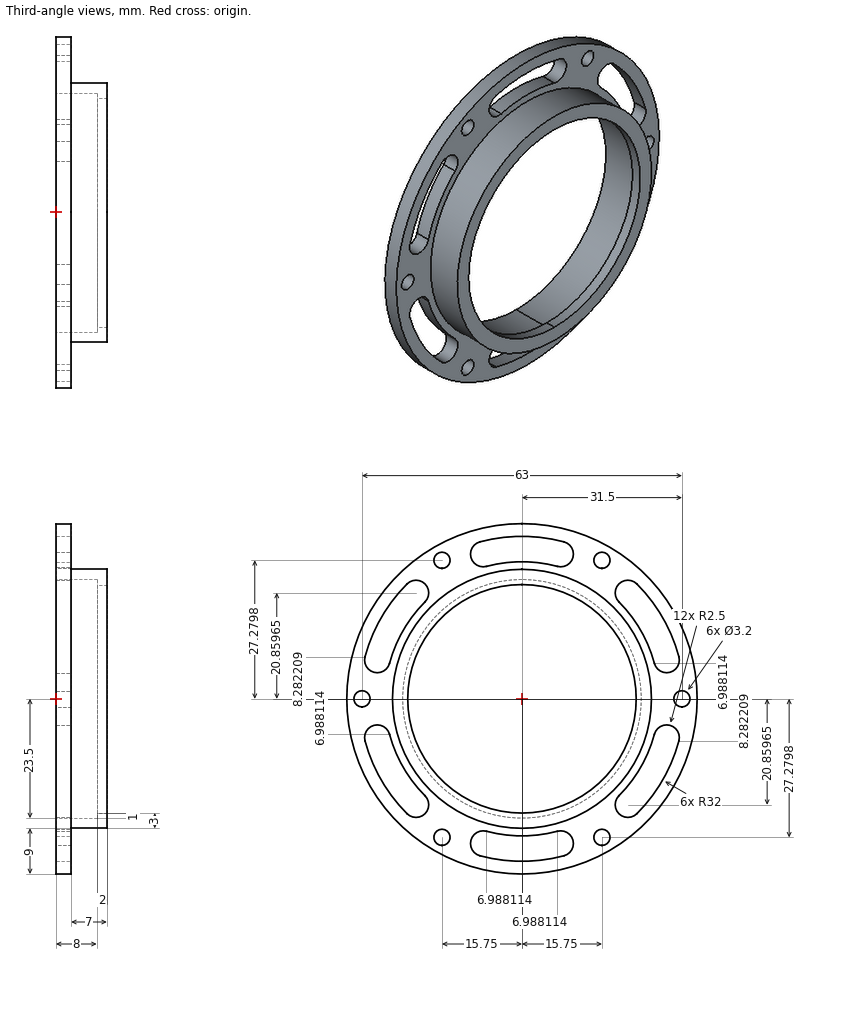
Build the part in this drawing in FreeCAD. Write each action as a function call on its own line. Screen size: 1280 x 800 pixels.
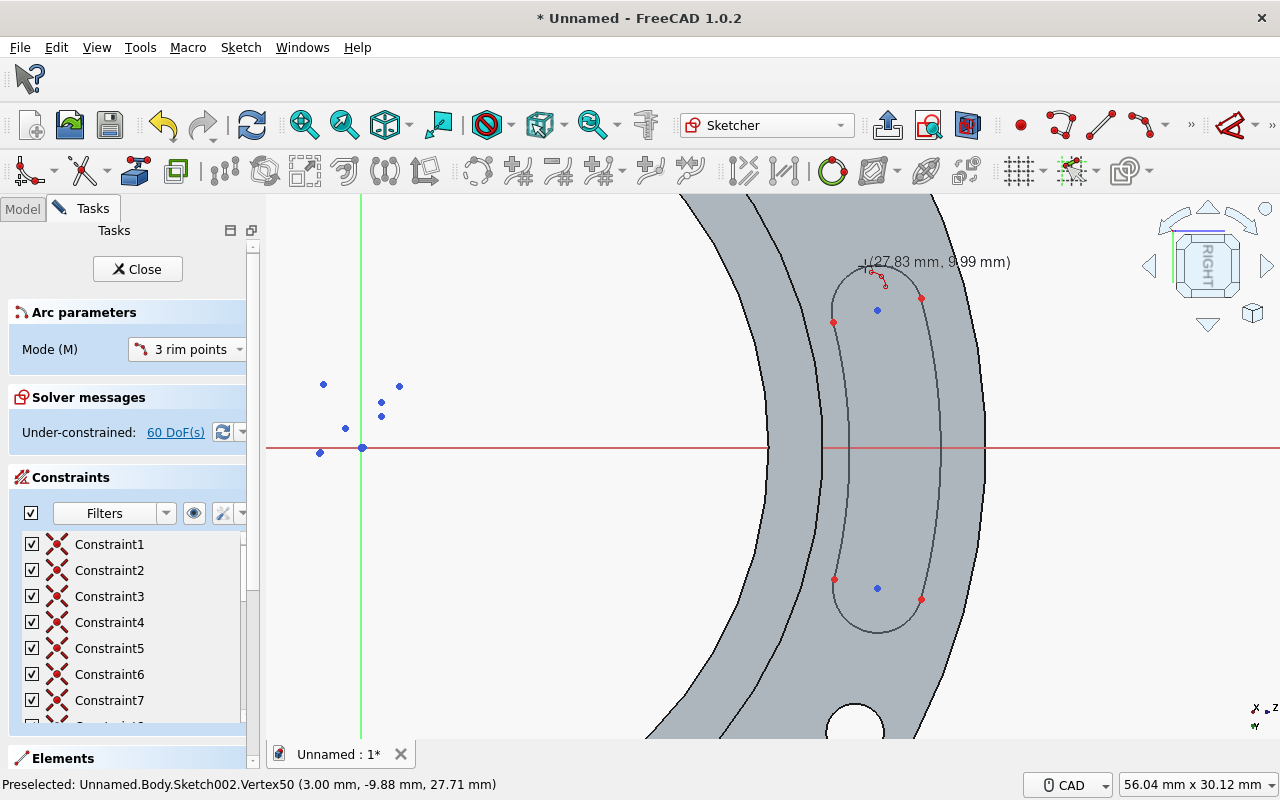
scroll(852, 475, down, 6)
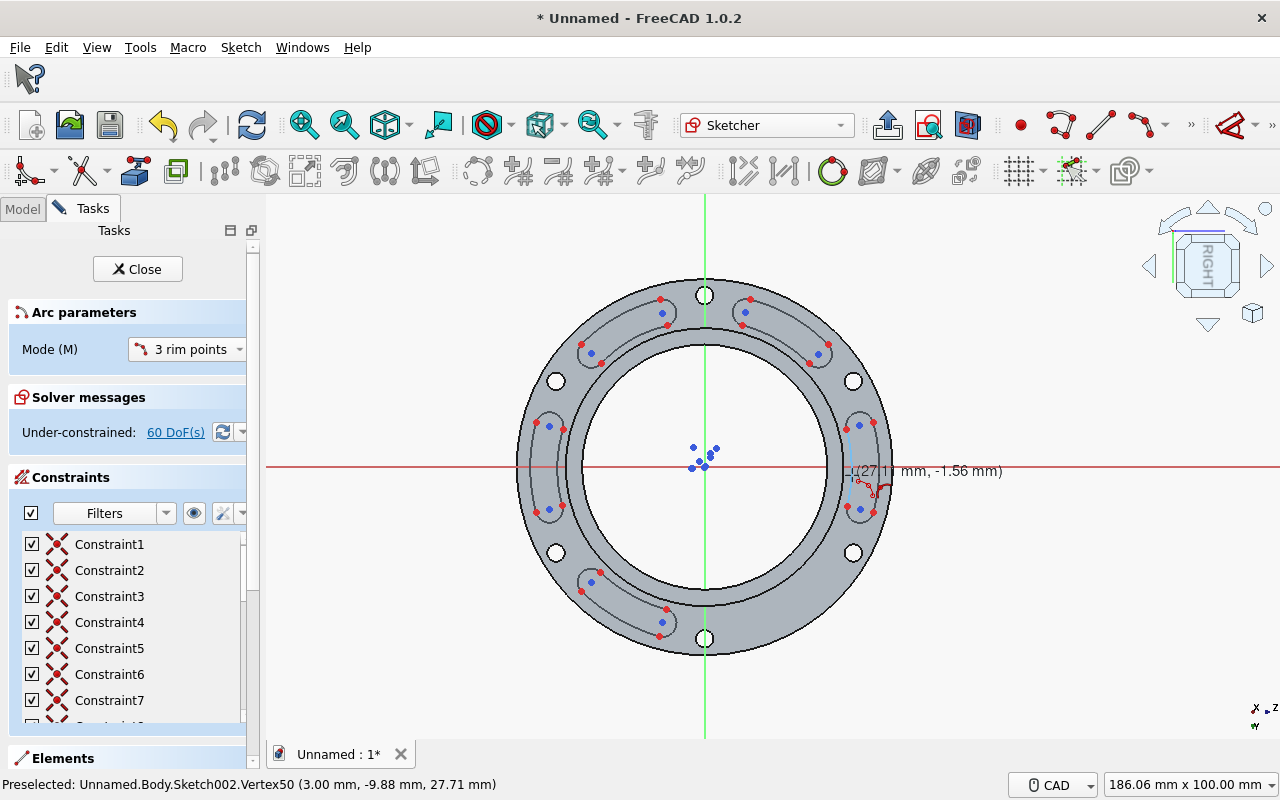
click(809, 571)
click(743, 609)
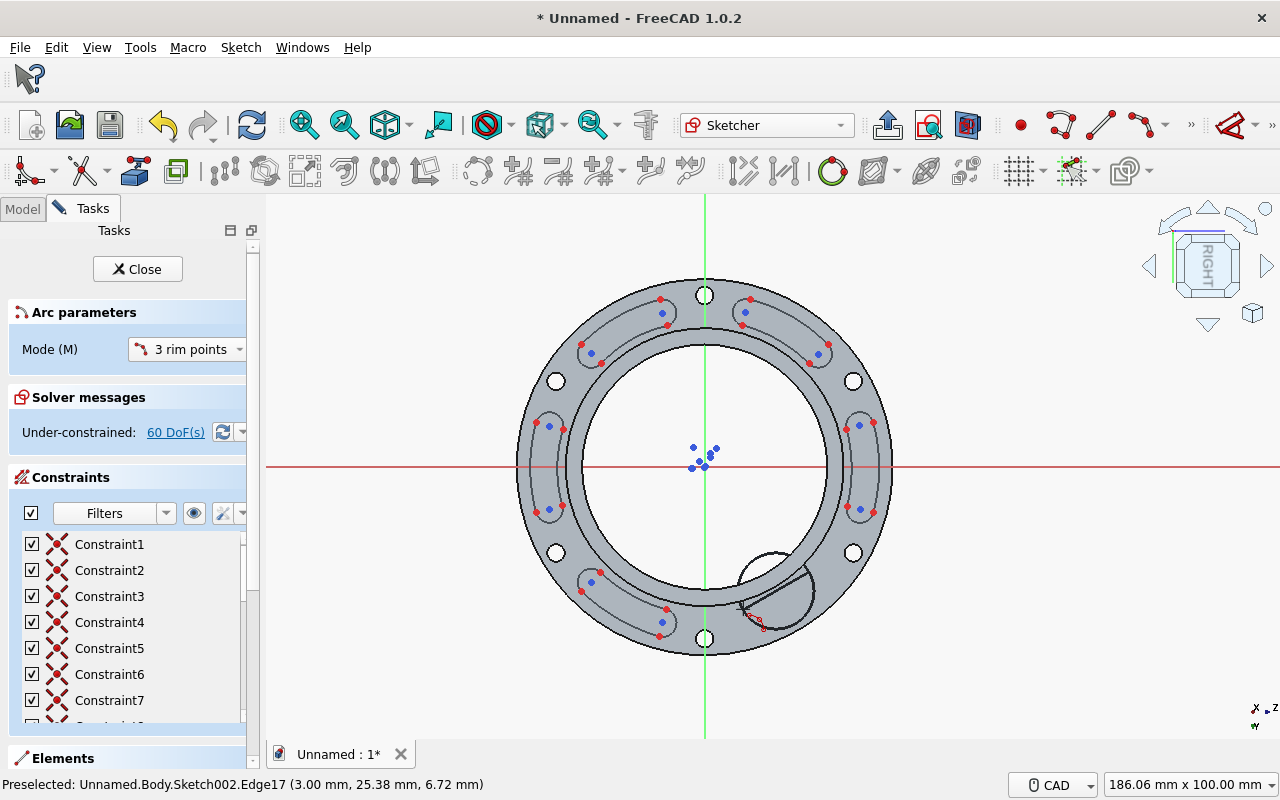
scroll(778, 595, up, 6)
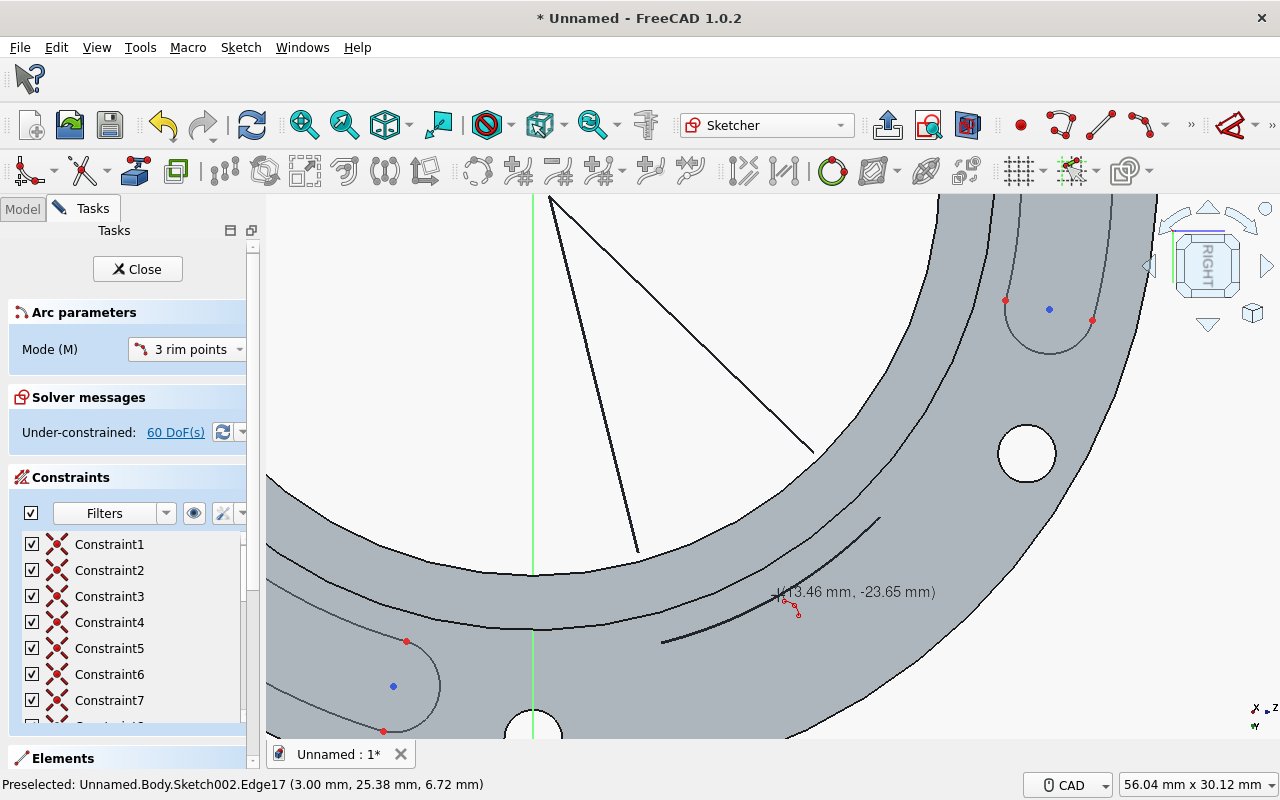
click(778, 592)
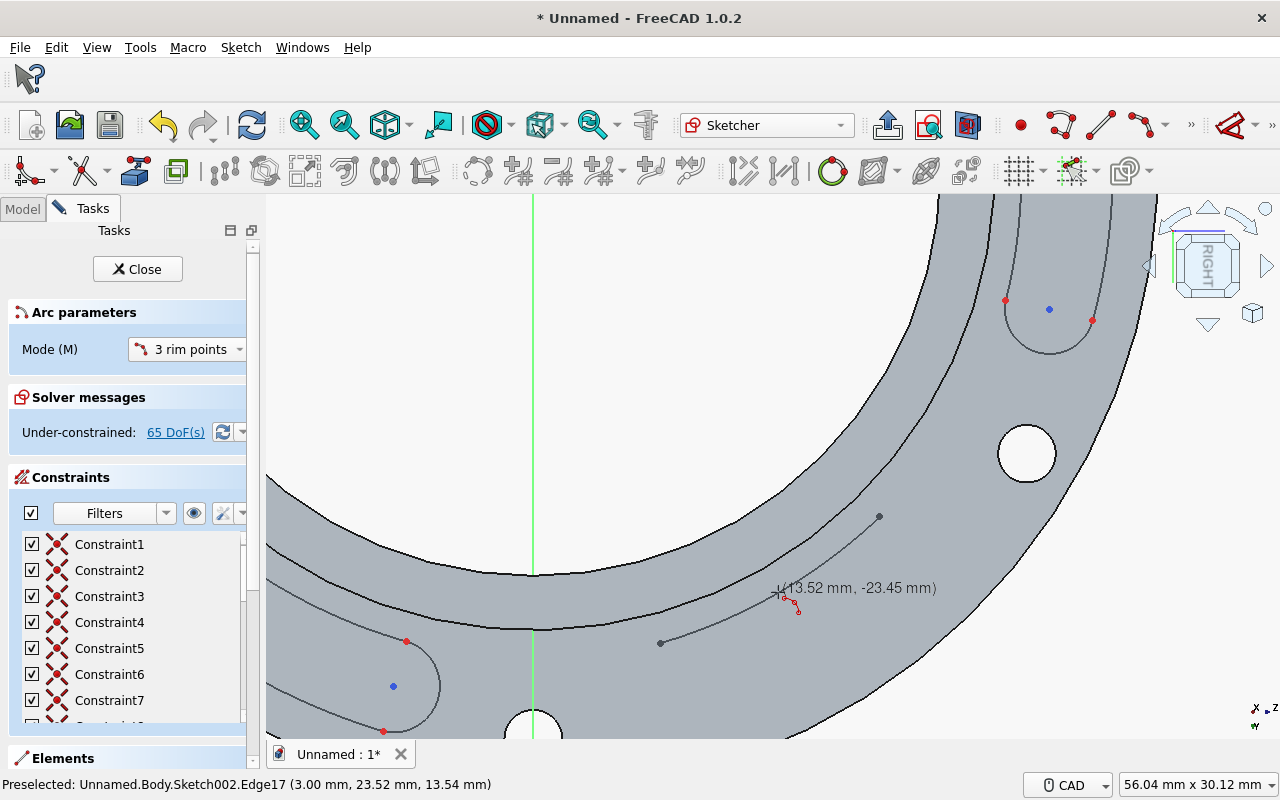
click(661, 643)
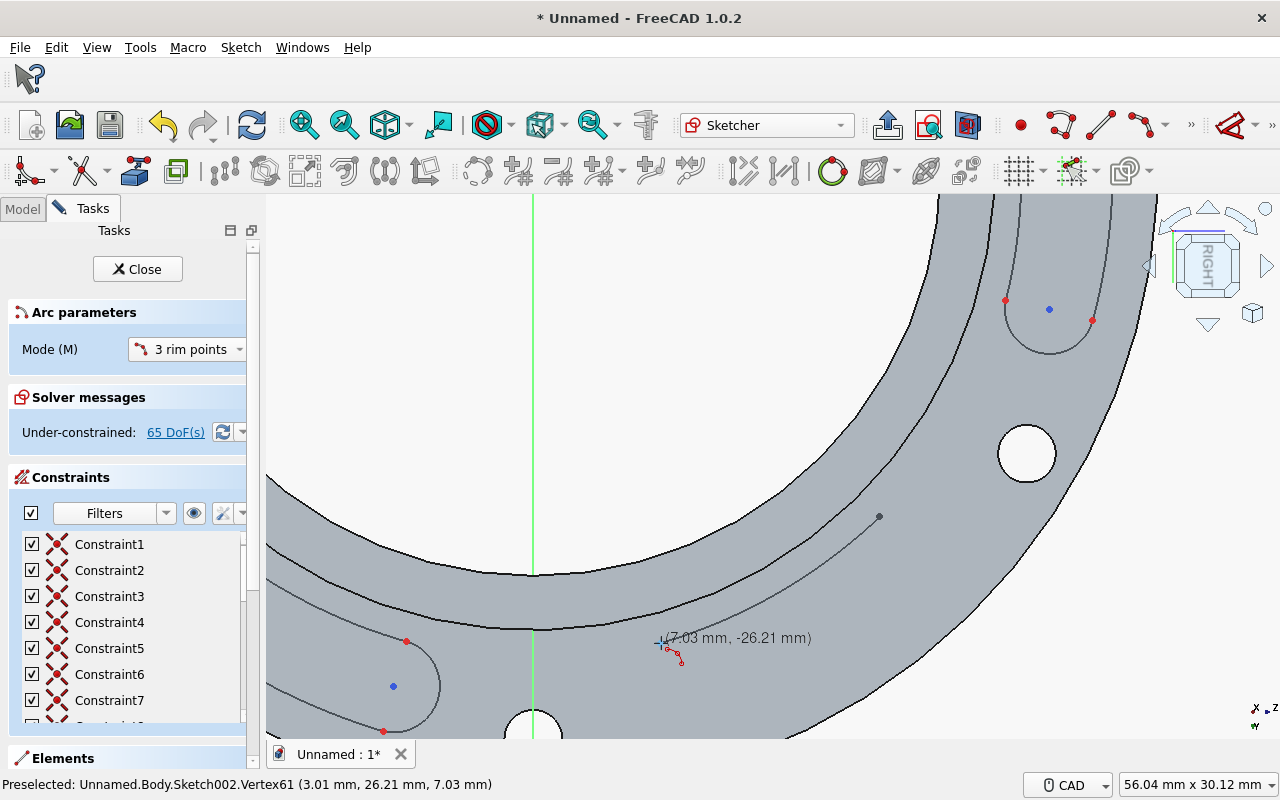
scroll(778, 595, down, 6)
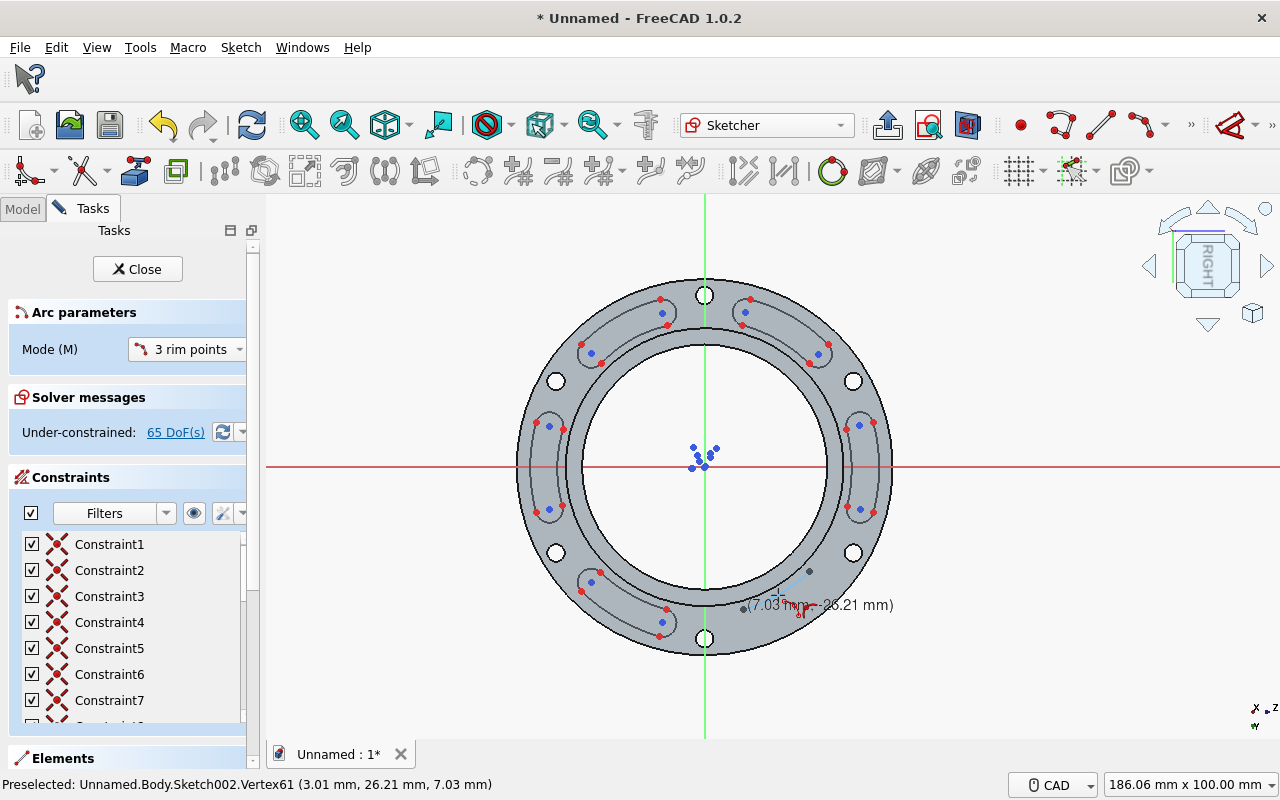
click(750, 636)
click(733, 626)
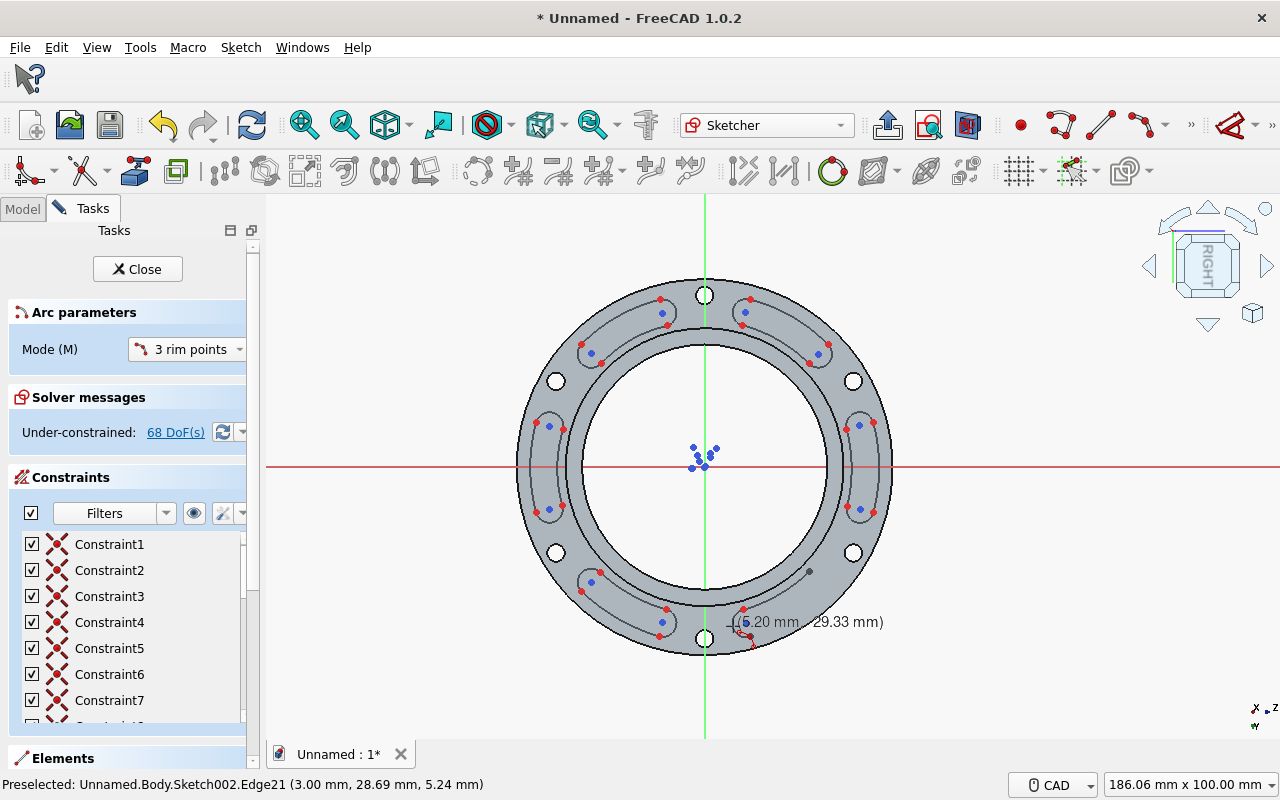
click(750, 637)
click(828, 590)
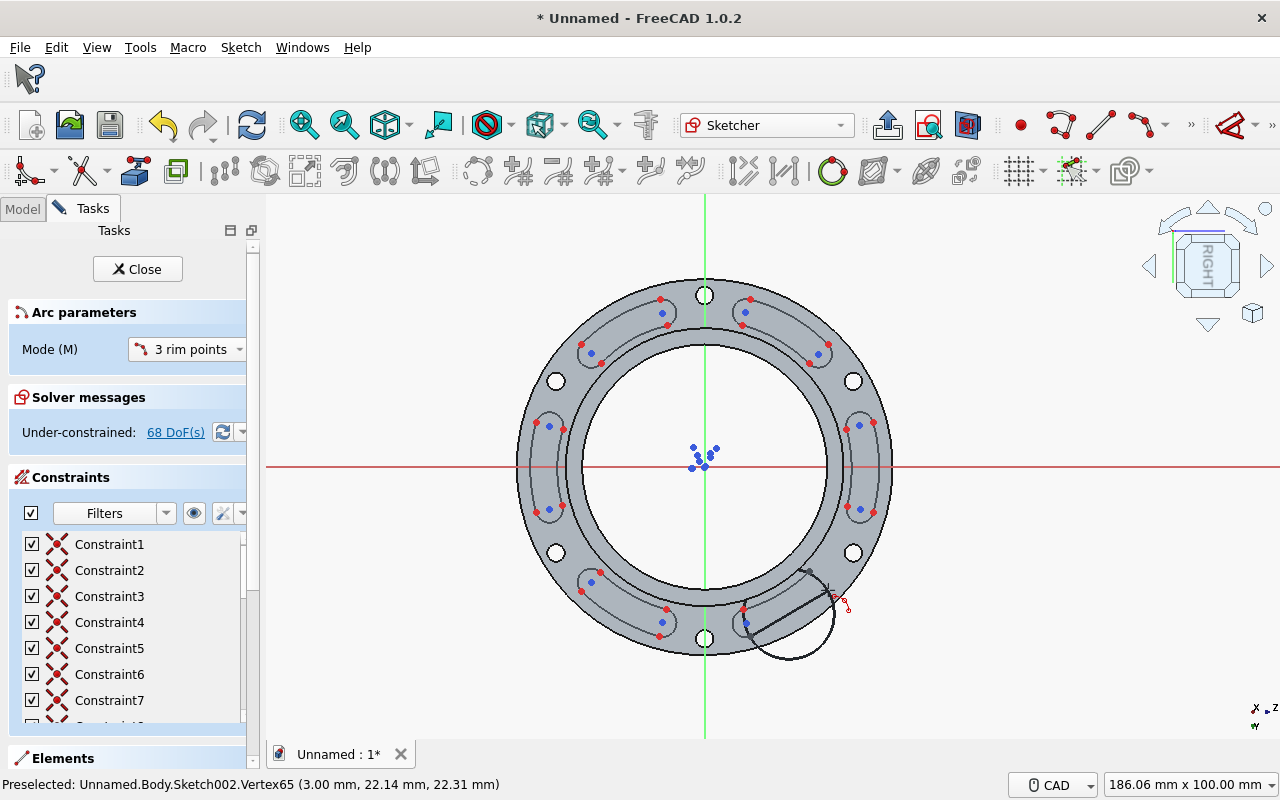
scroll(792, 618, up, 5)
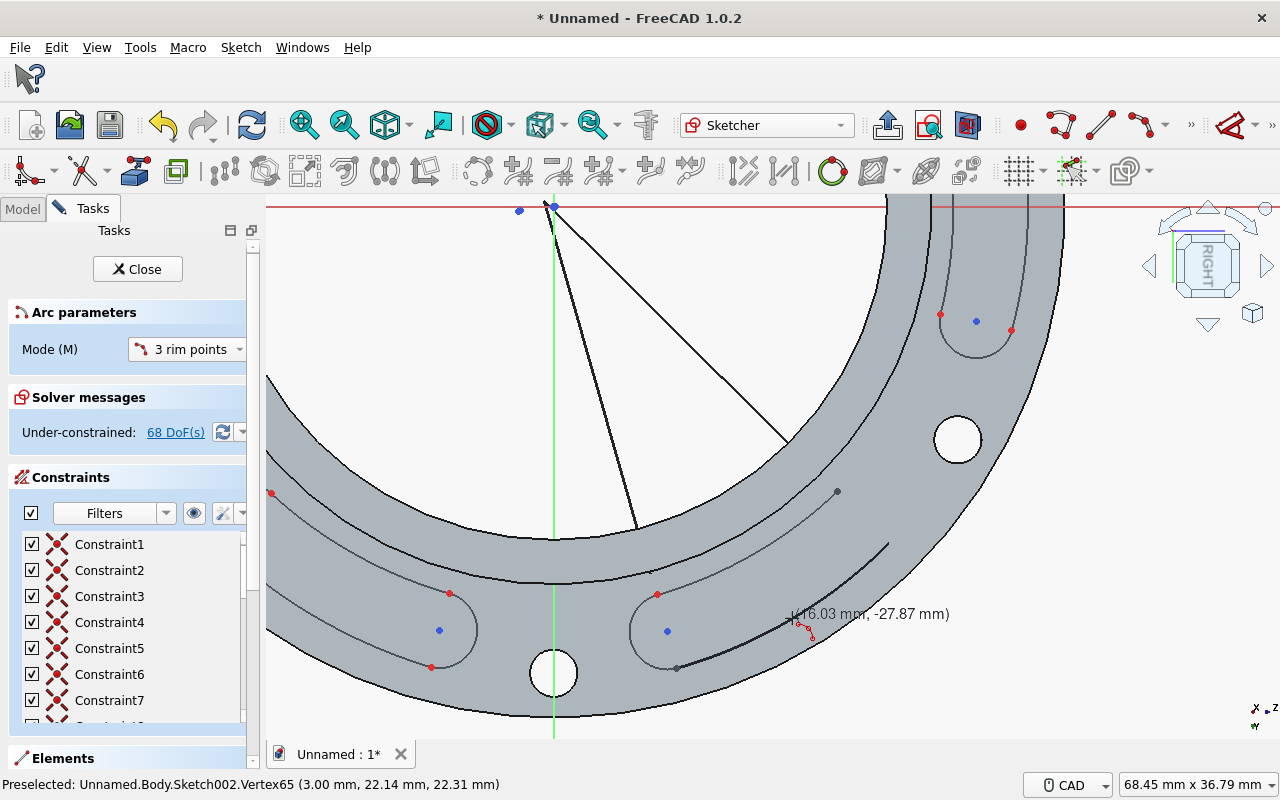
click(791, 617)